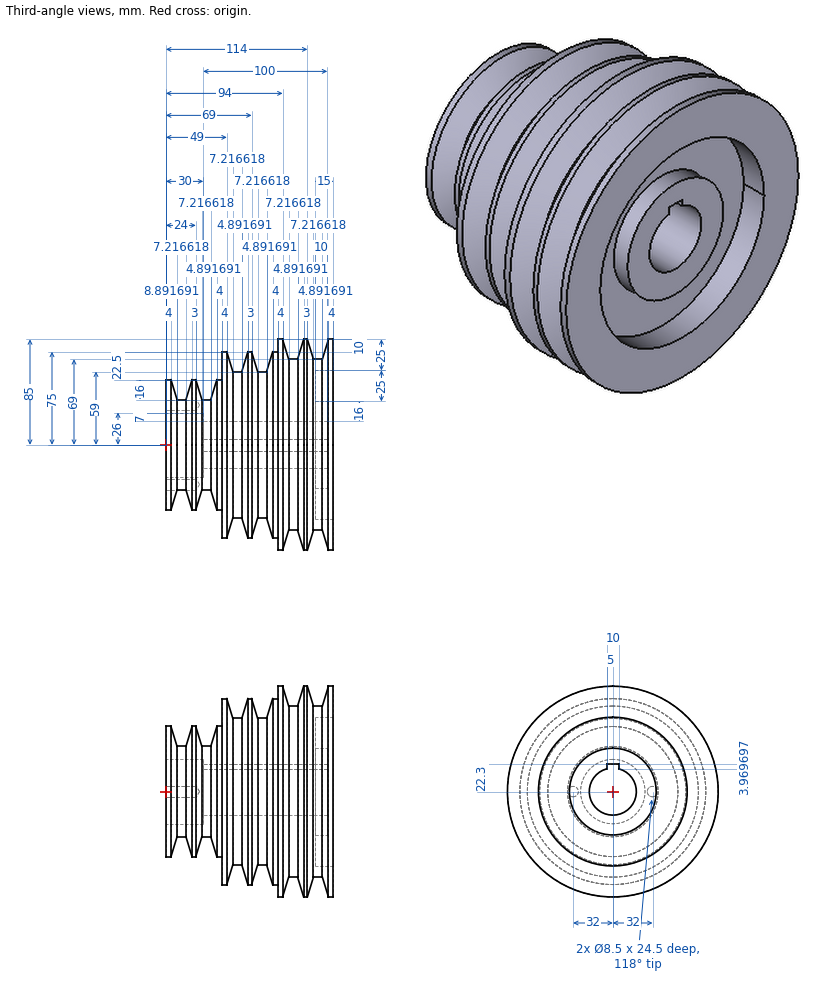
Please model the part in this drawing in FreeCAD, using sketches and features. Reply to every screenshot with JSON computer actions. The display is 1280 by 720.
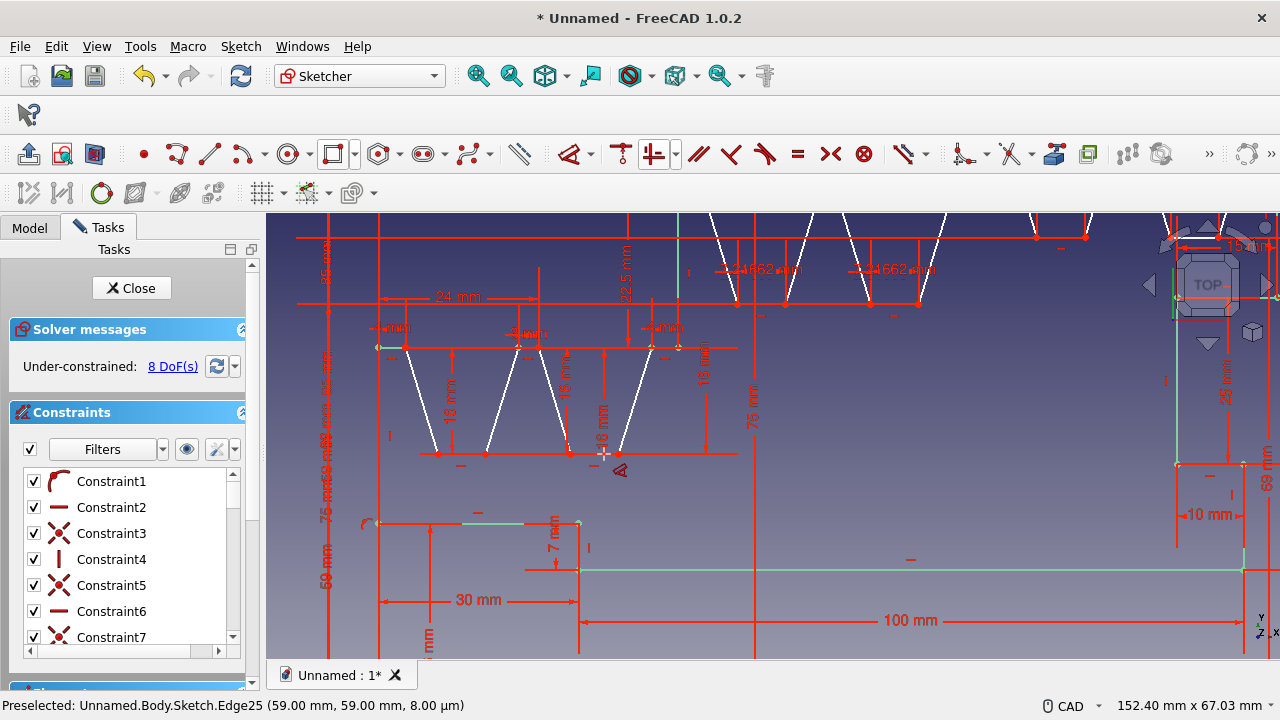
{"action": "left_click", "coordinate": [604, 454]}
{"action": "left_click", "coordinate": [595, 488]}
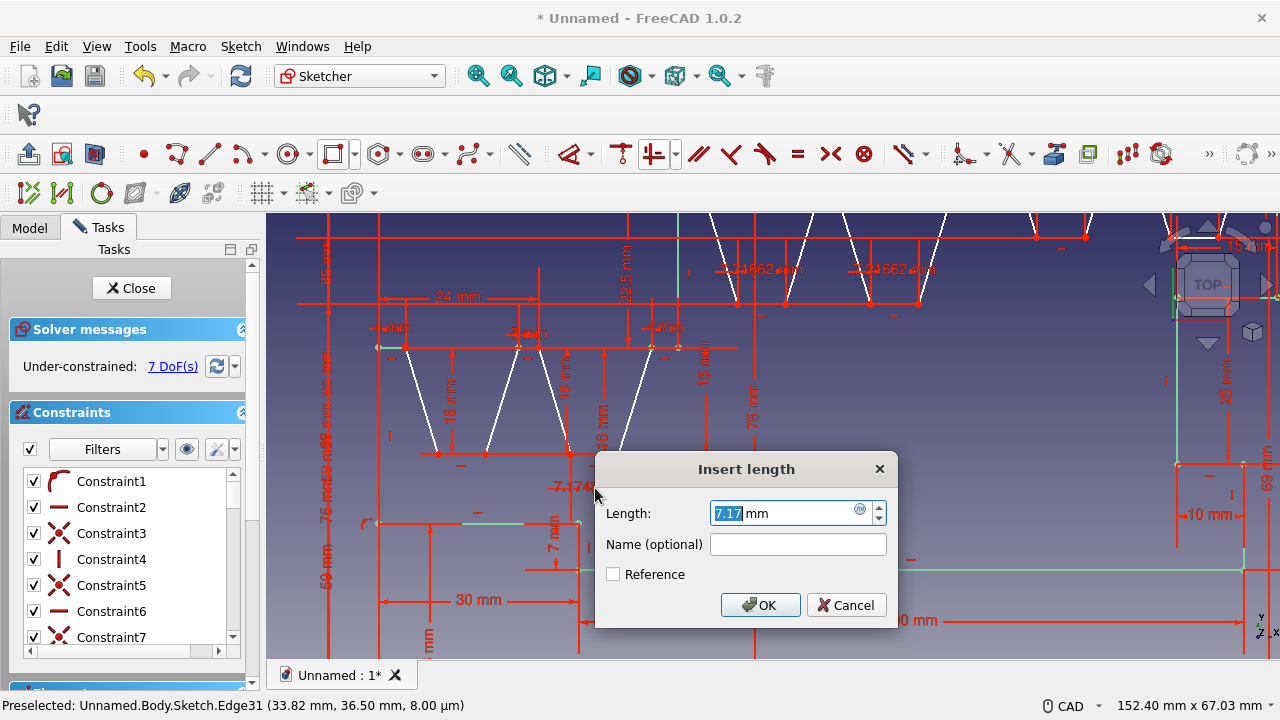
{"action": "type", "text": "7.216618"}
{"action": "key", "text": "Return"}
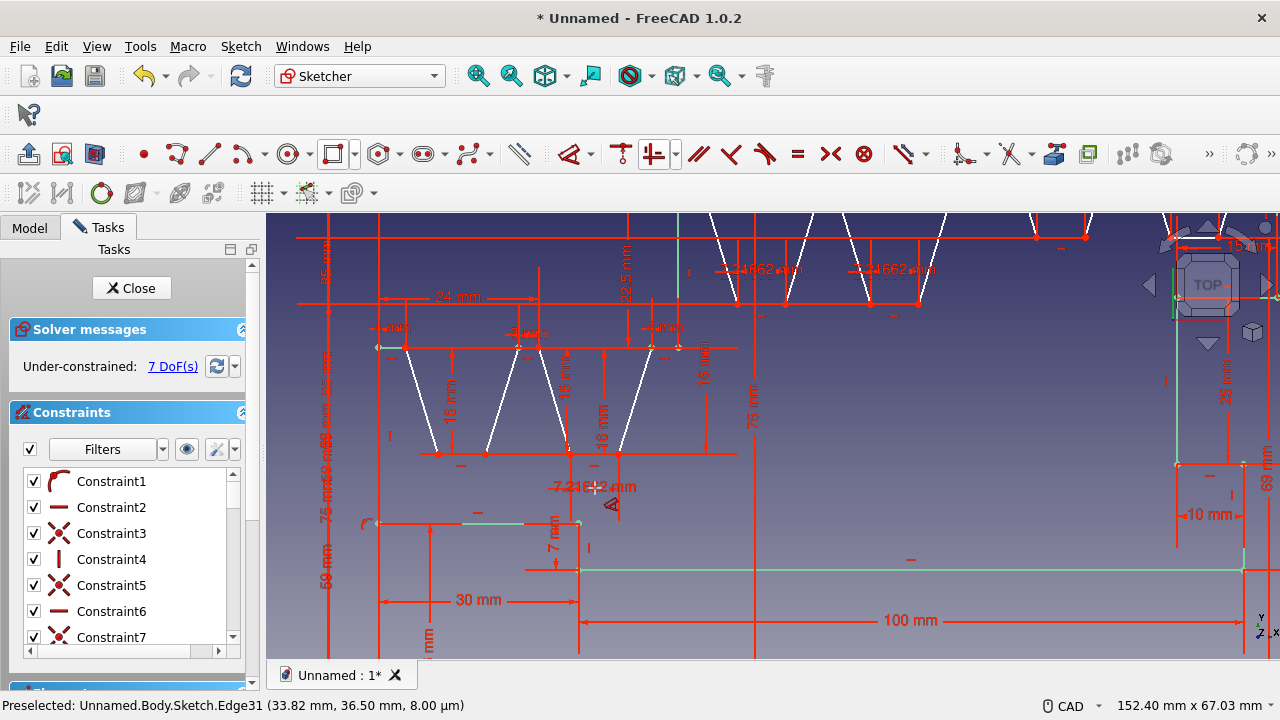
{"action": "left_click", "coordinate": [471, 454]}
{"action": "left_click", "coordinate": [462, 488]}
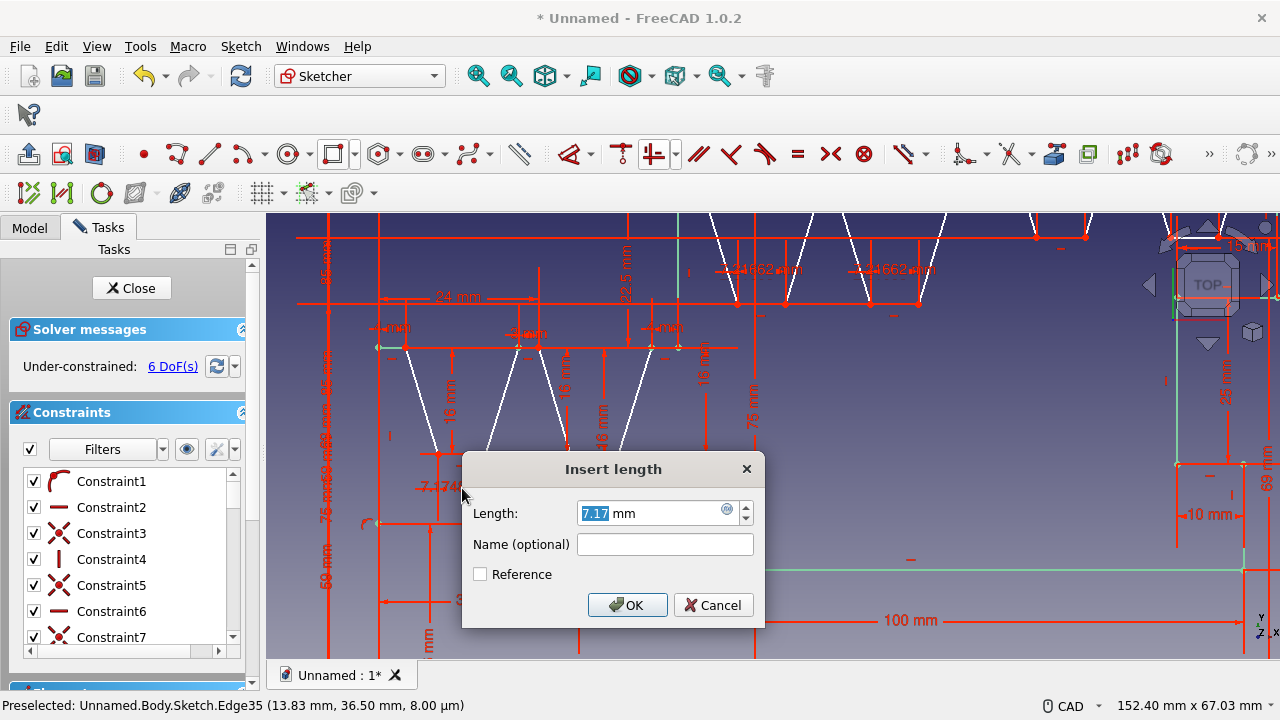
{"action": "type", "text": "7.216618"}
{"action": "key", "text": "Return"}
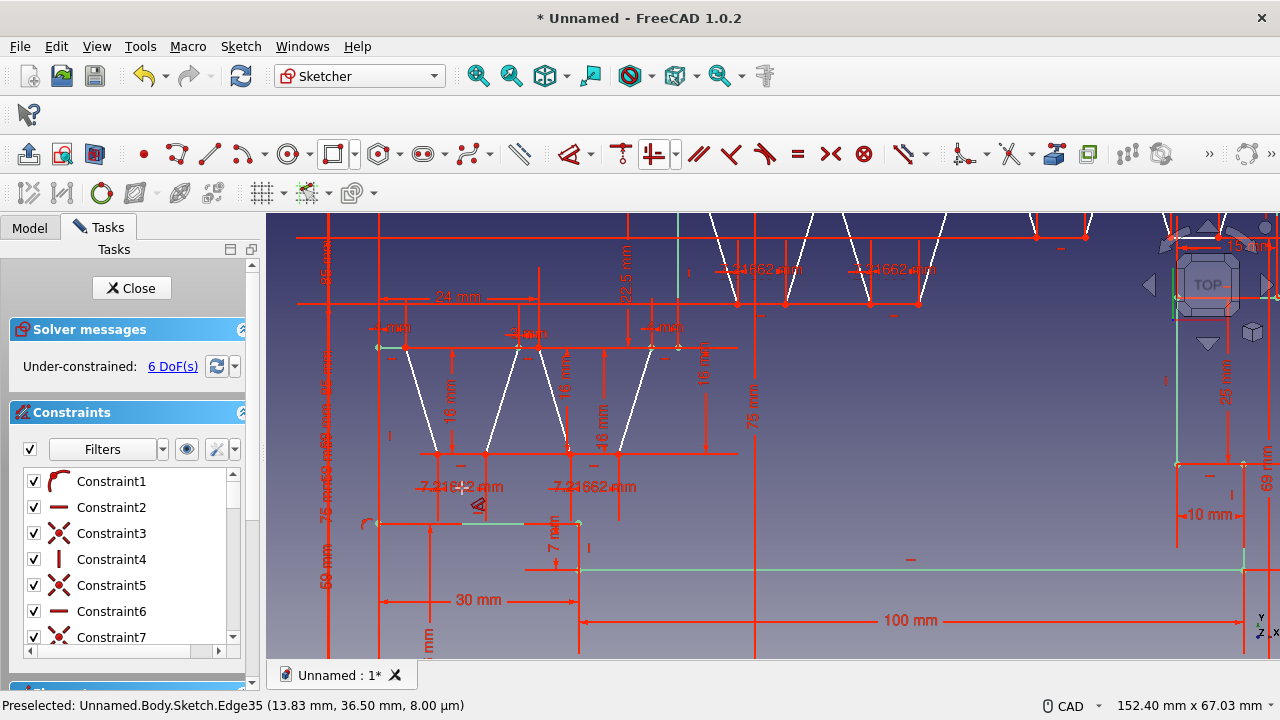
{"action": "left_click", "coordinate": [438, 454]}
{"action": "left_click", "coordinate": [429, 372]}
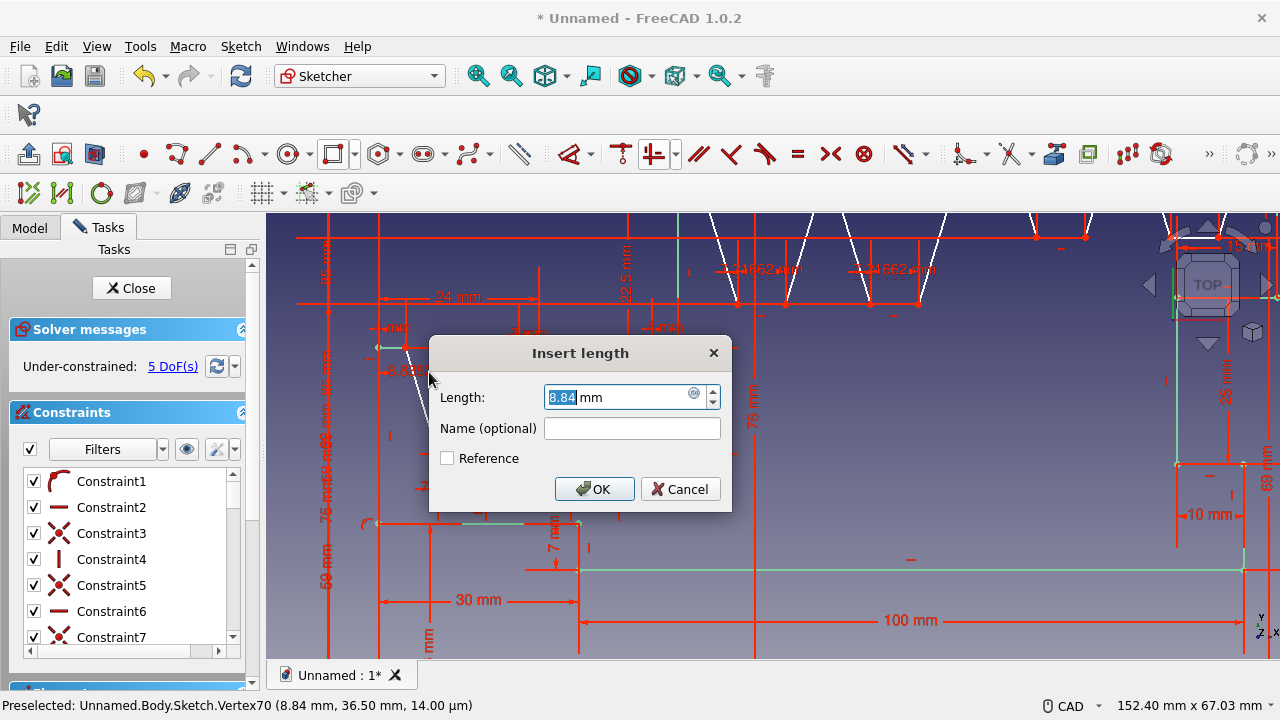
{"action": "type", "text": "8.891691"}
{"action": "key", "text": "Return"}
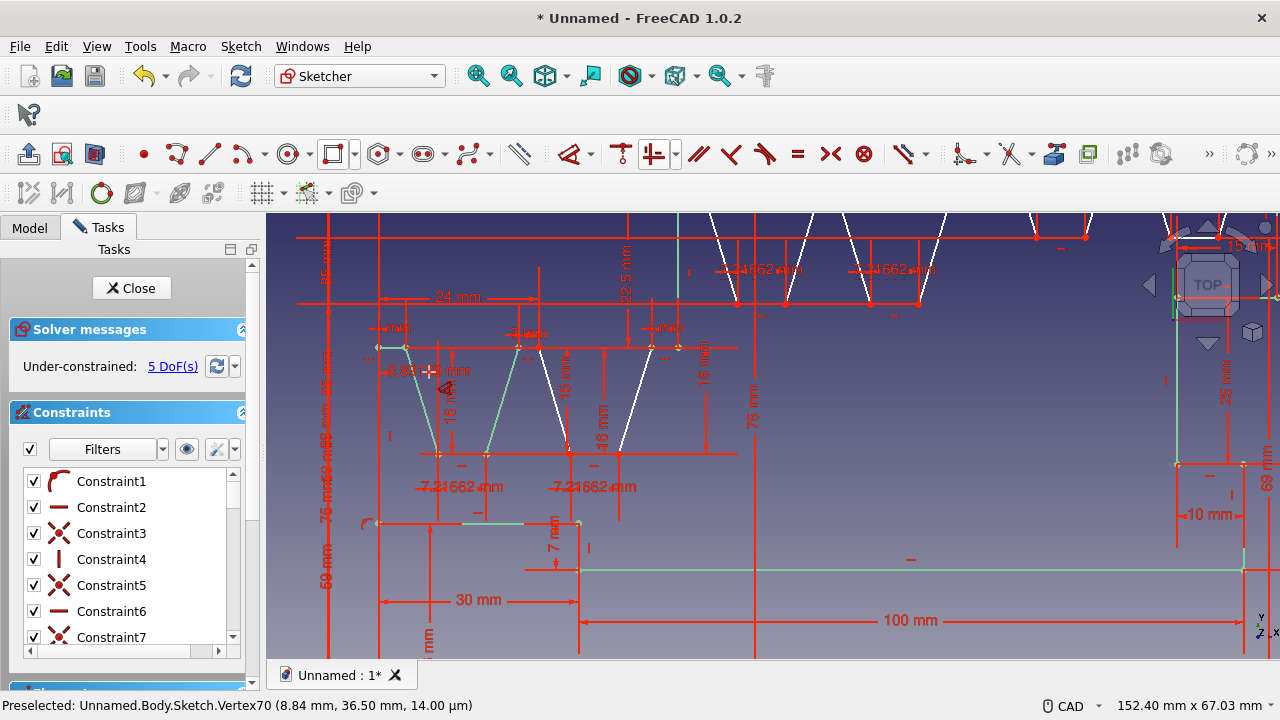
{"action": "scroll", "coordinate": [604, 454], "scroll_direction": "down", "scroll_amount": 4}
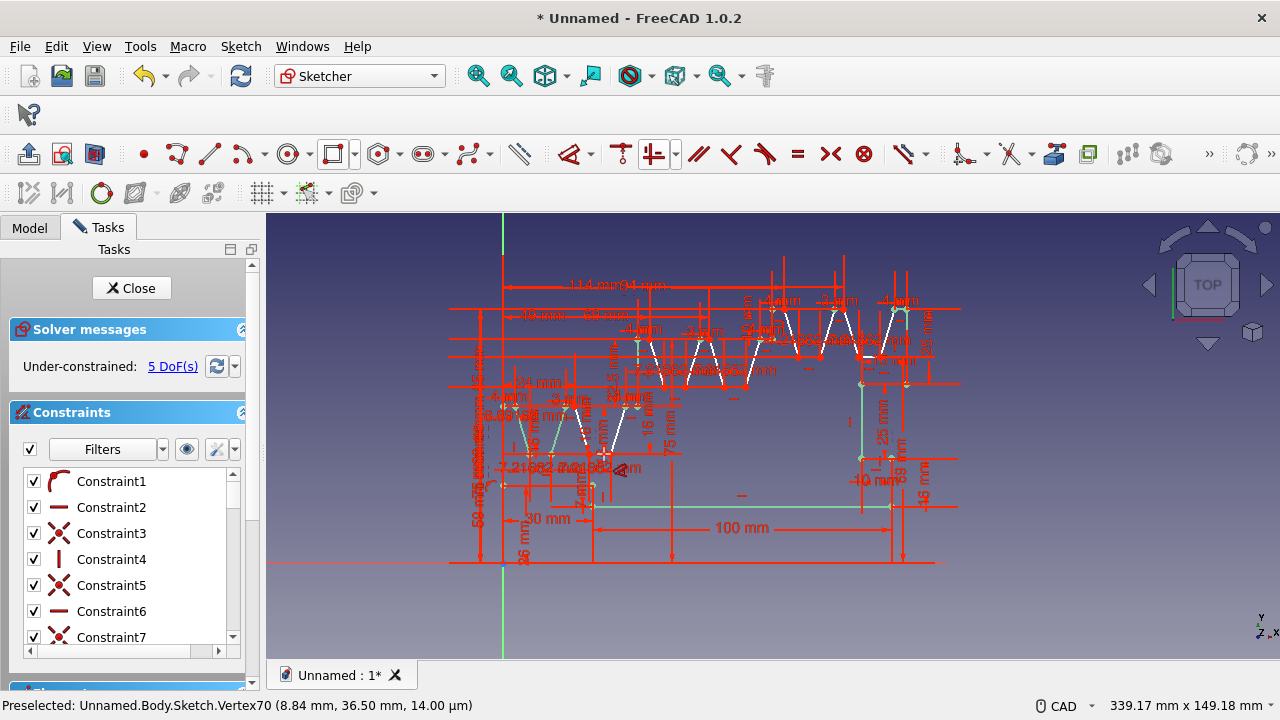
{"action": "scroll", "coordinate": [890, 324], "scroll_direction": "up", "scroll_amount": 5}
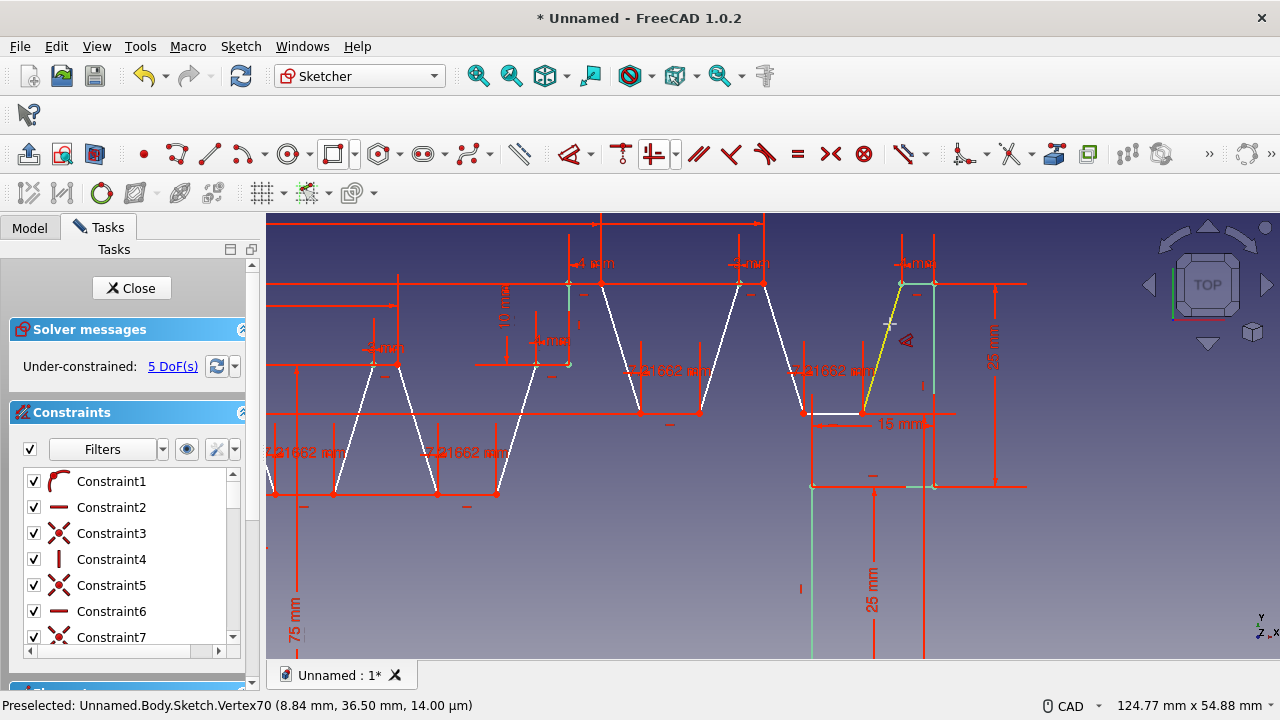
{"action": "left_click", "coordinate": [890, 323]}
{"action": "left_click", "coordinate": [882, 472]}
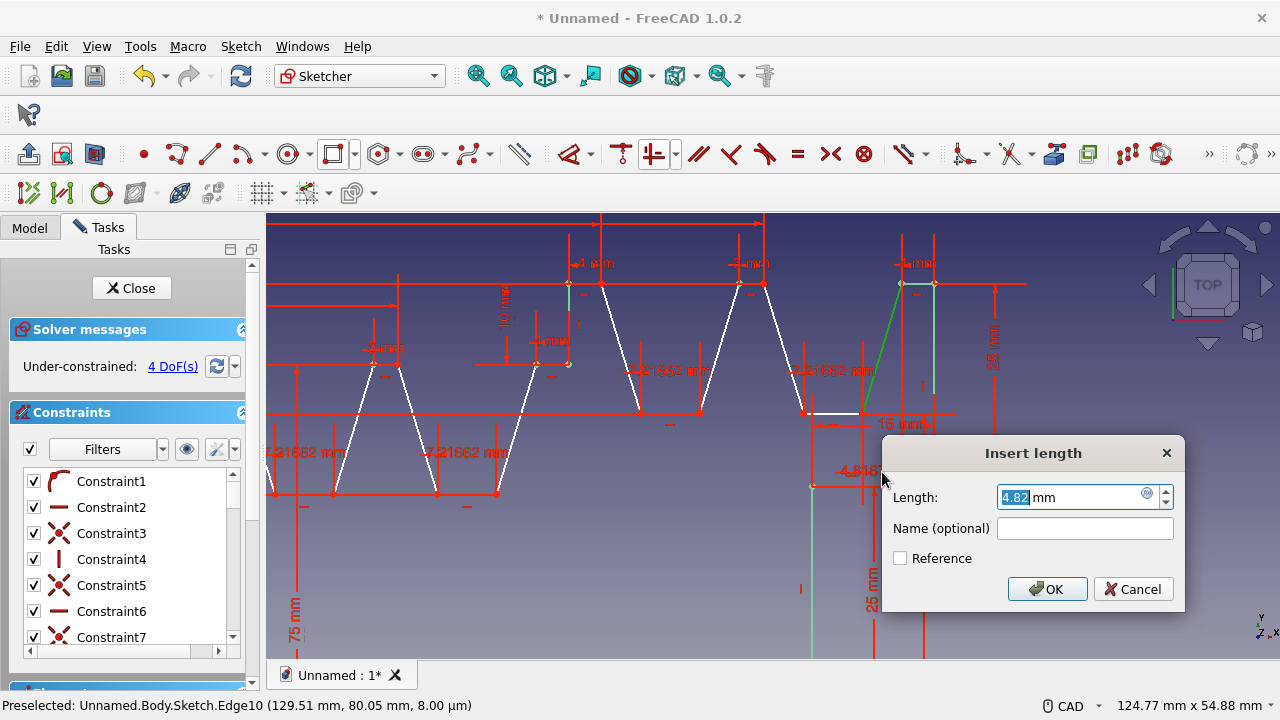
{"action": "type", "text": "4.891691"}
{"action": "key", "text": "Return"}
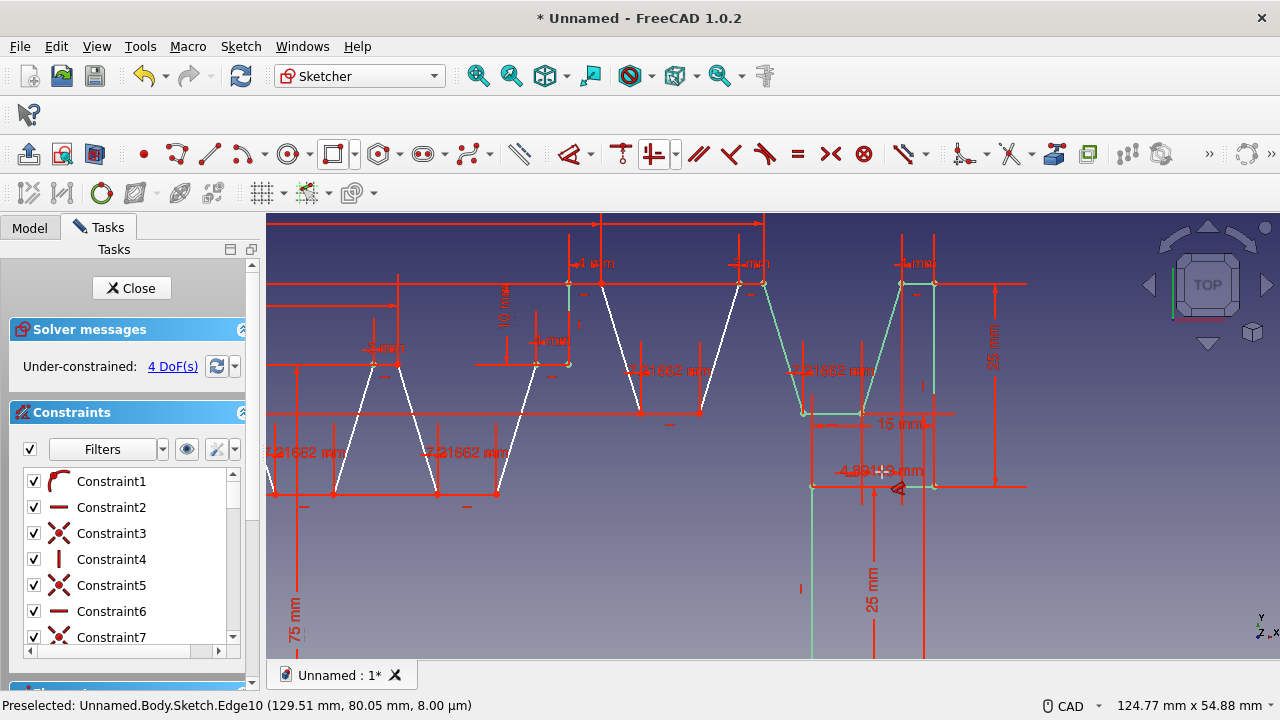
{"action": "left_click", "coordinate": [727, 323]}
{"action": "left_click", "coordinate": [719, 448]}